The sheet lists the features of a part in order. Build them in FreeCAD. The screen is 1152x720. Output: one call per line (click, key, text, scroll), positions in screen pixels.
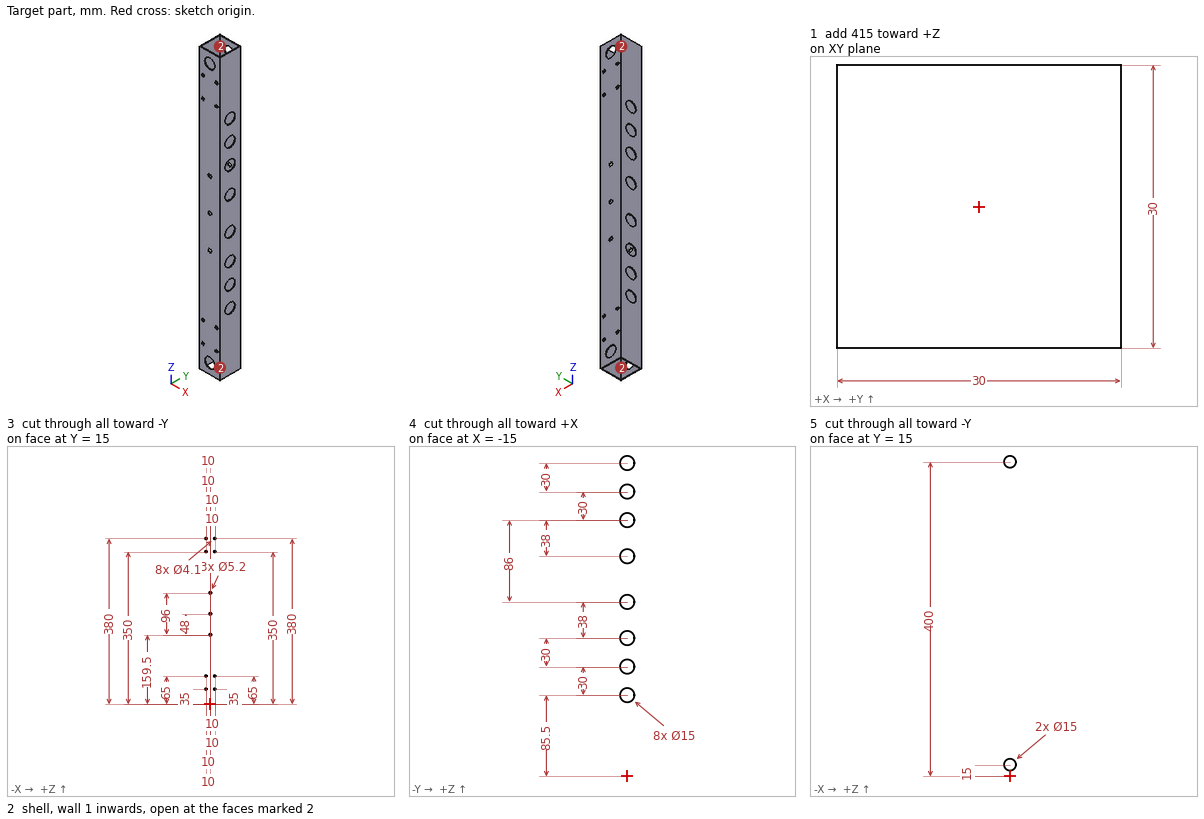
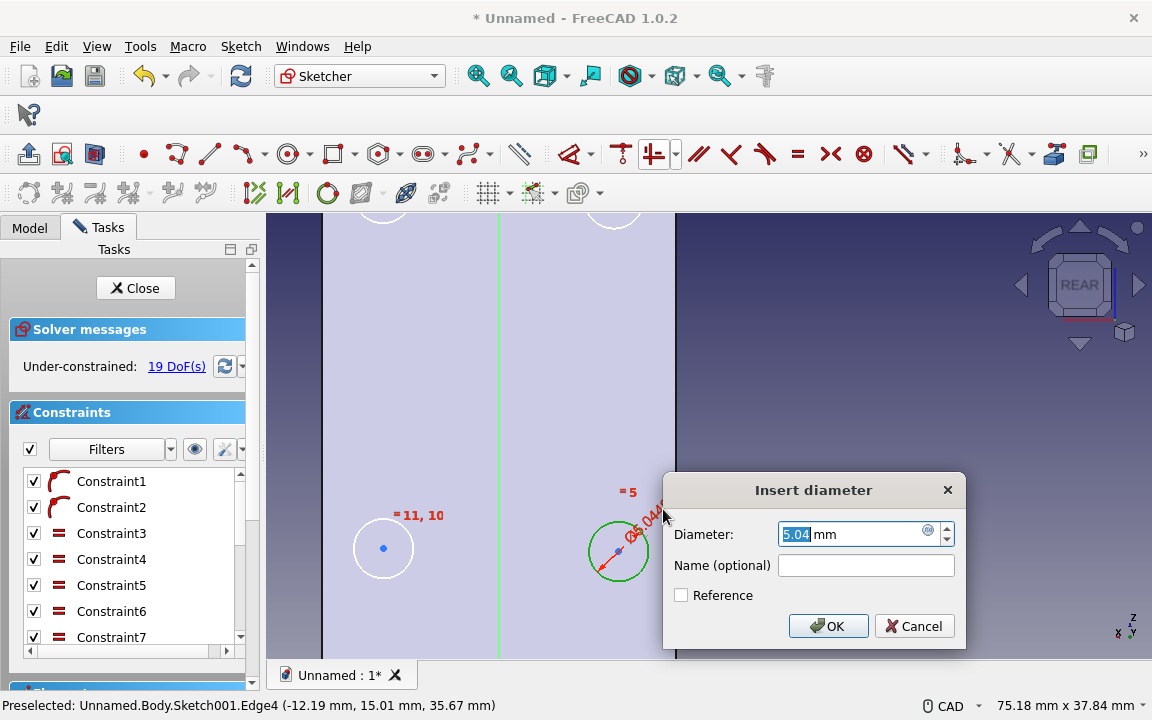
text(4.1)
key(Return)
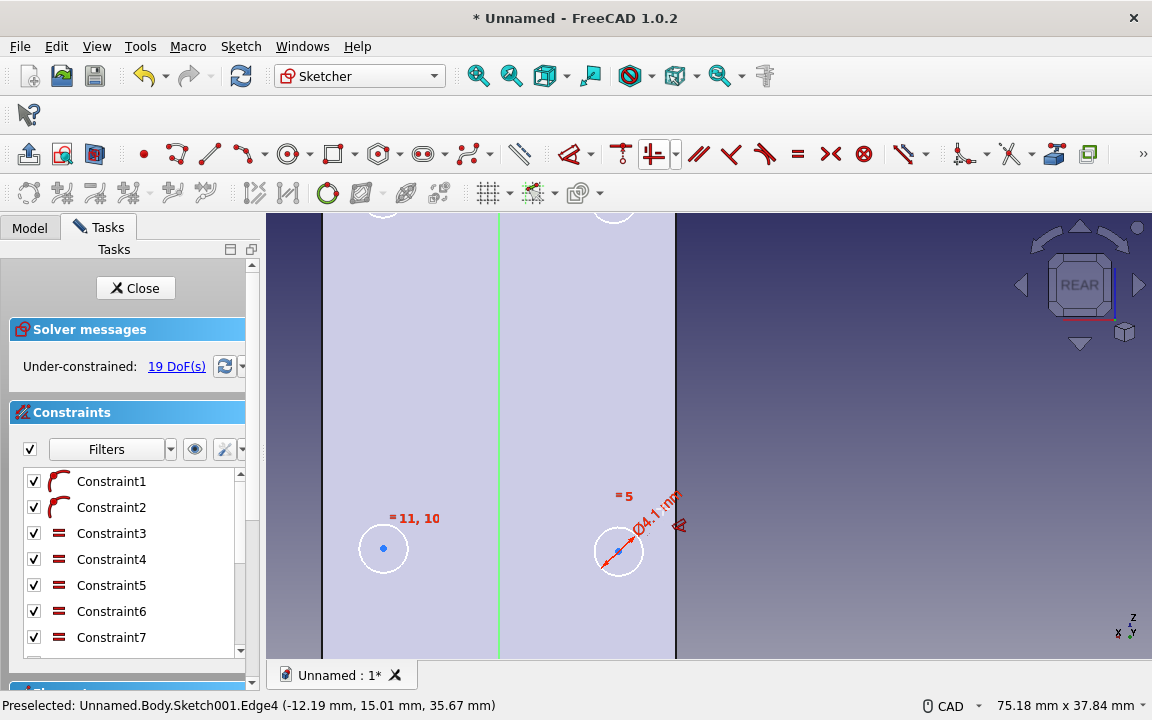
scroll(650, 548, down, 14)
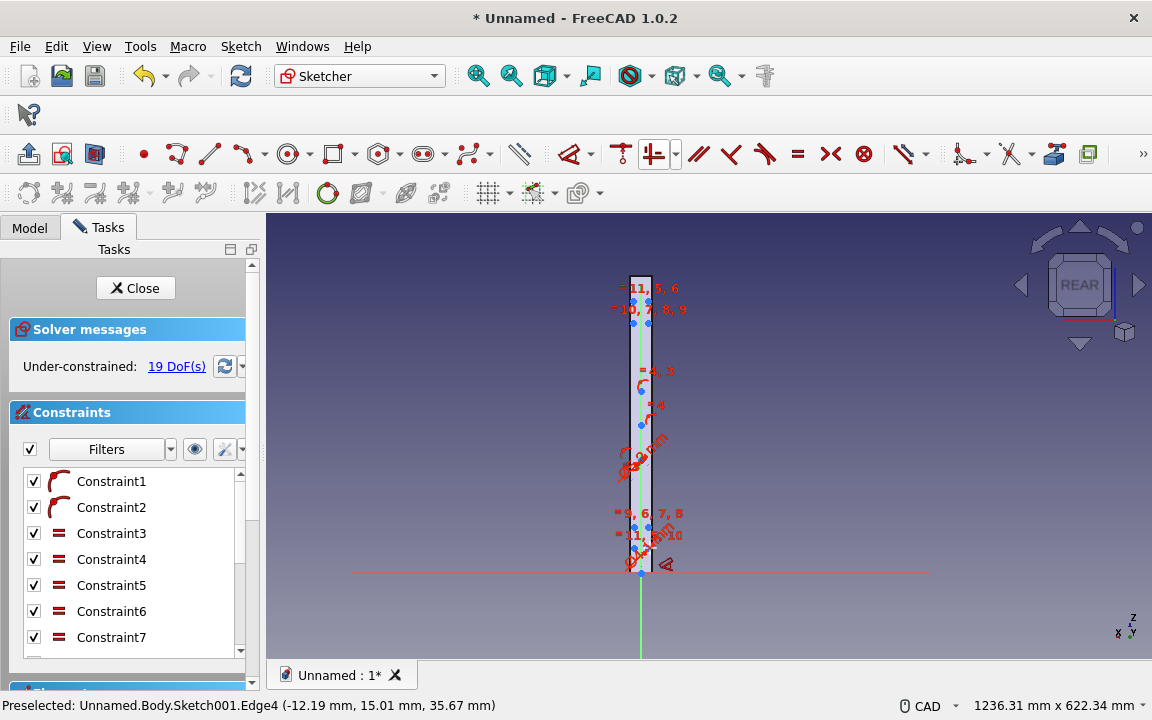
scroll(649, 549, up, 9)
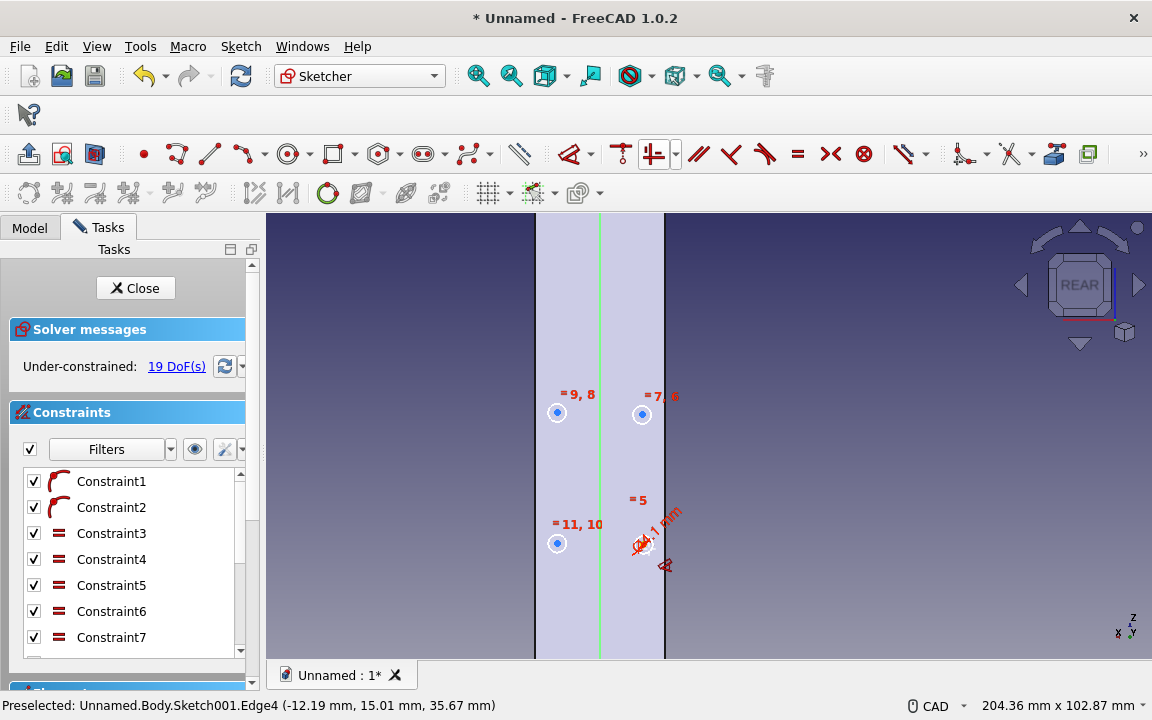
click(644, 545)
click(622, 487)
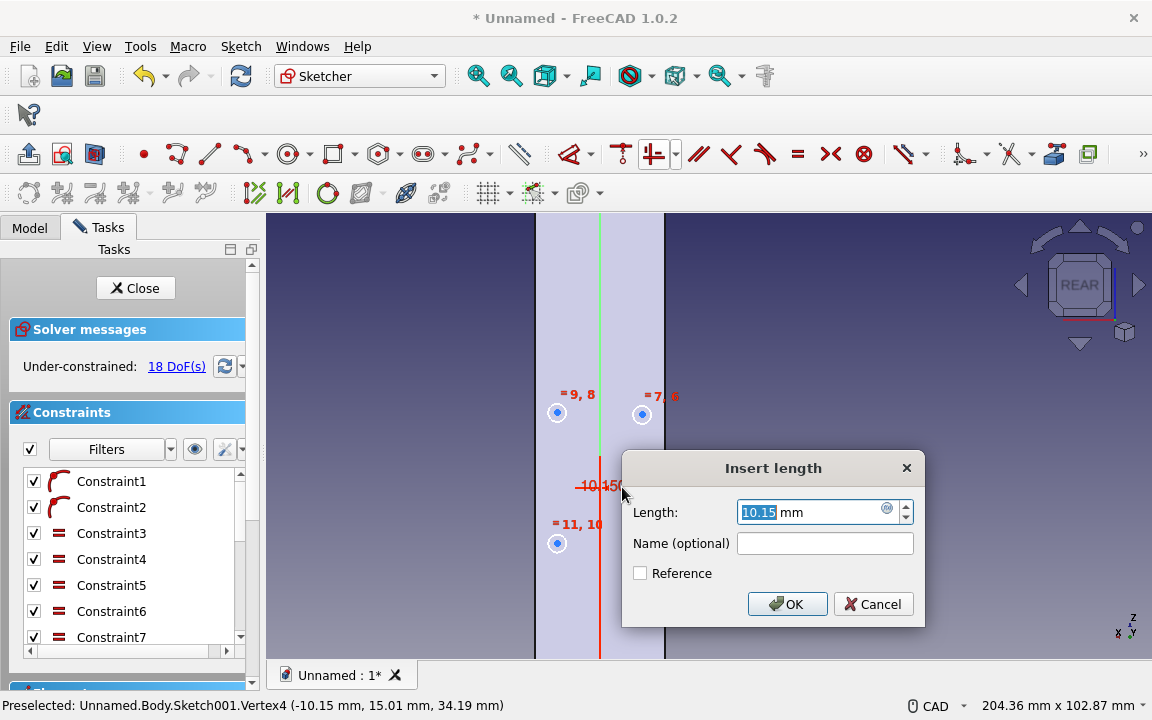
text(10)
key(Return)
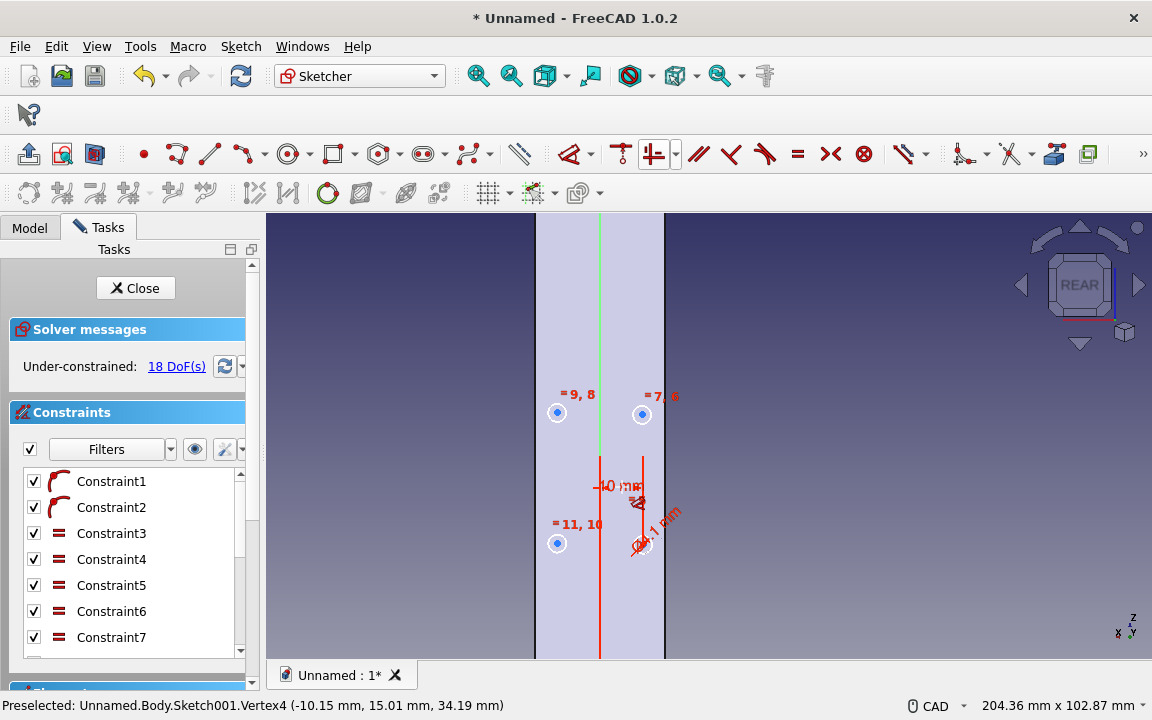
scroll(649, 549, down, 9)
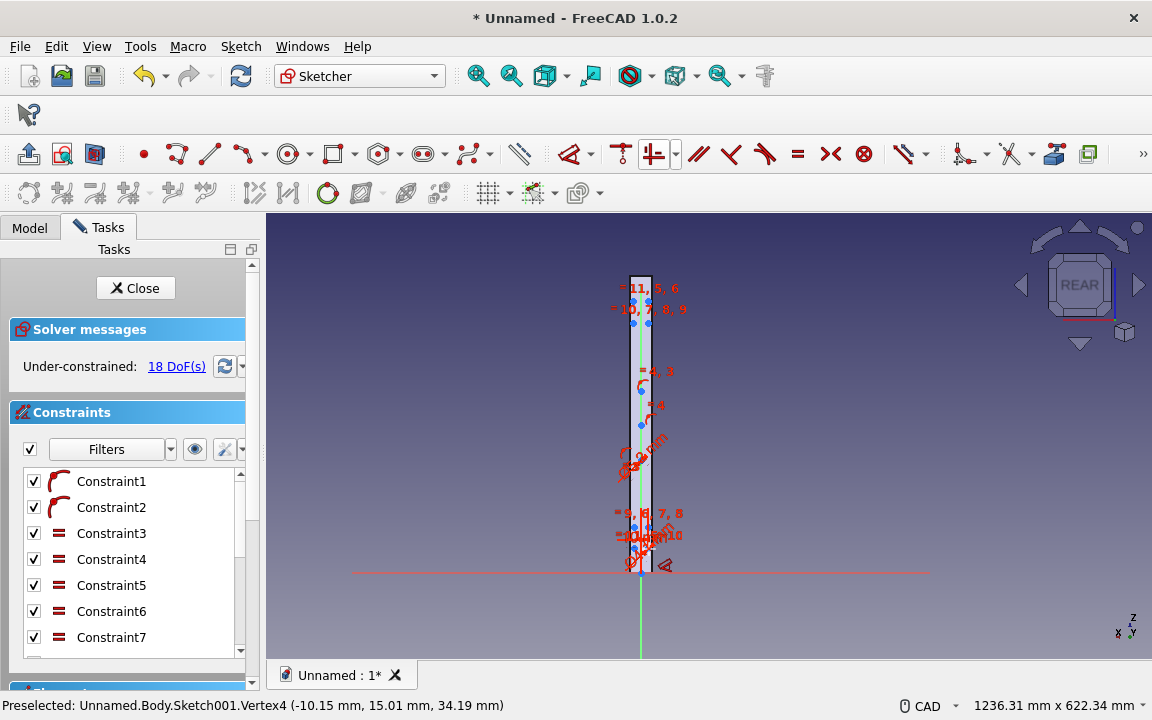
scroll(648, 549, up, 3)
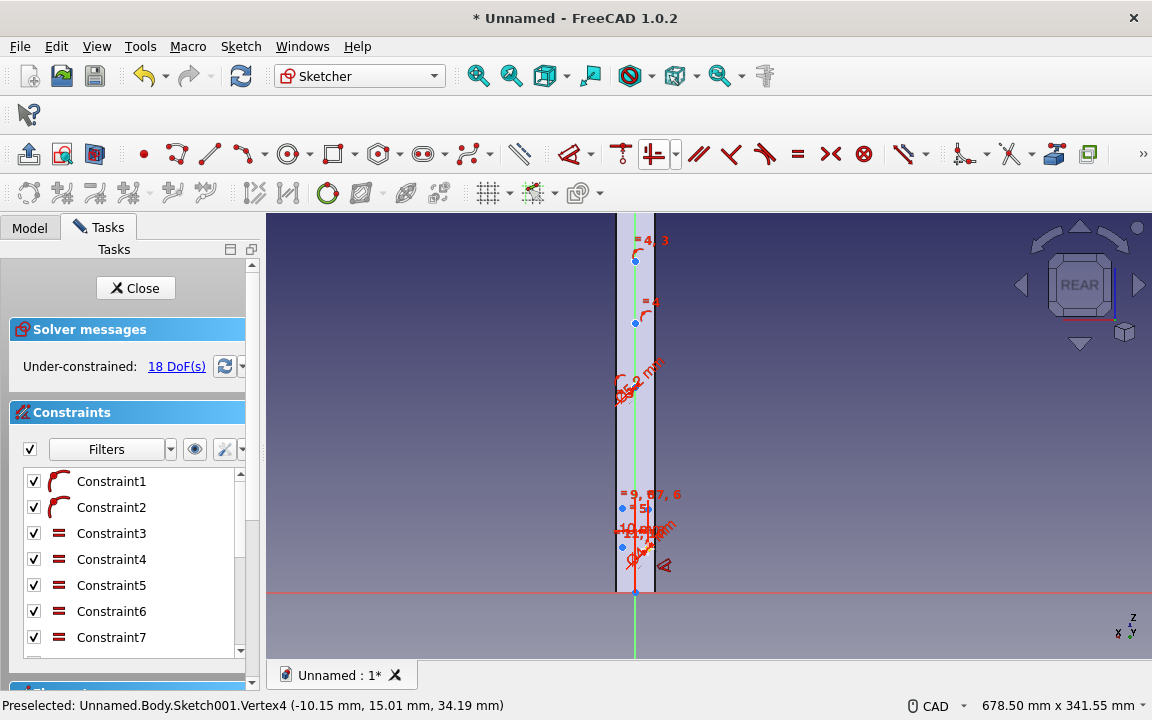
click(648, 548)
click(682, 571)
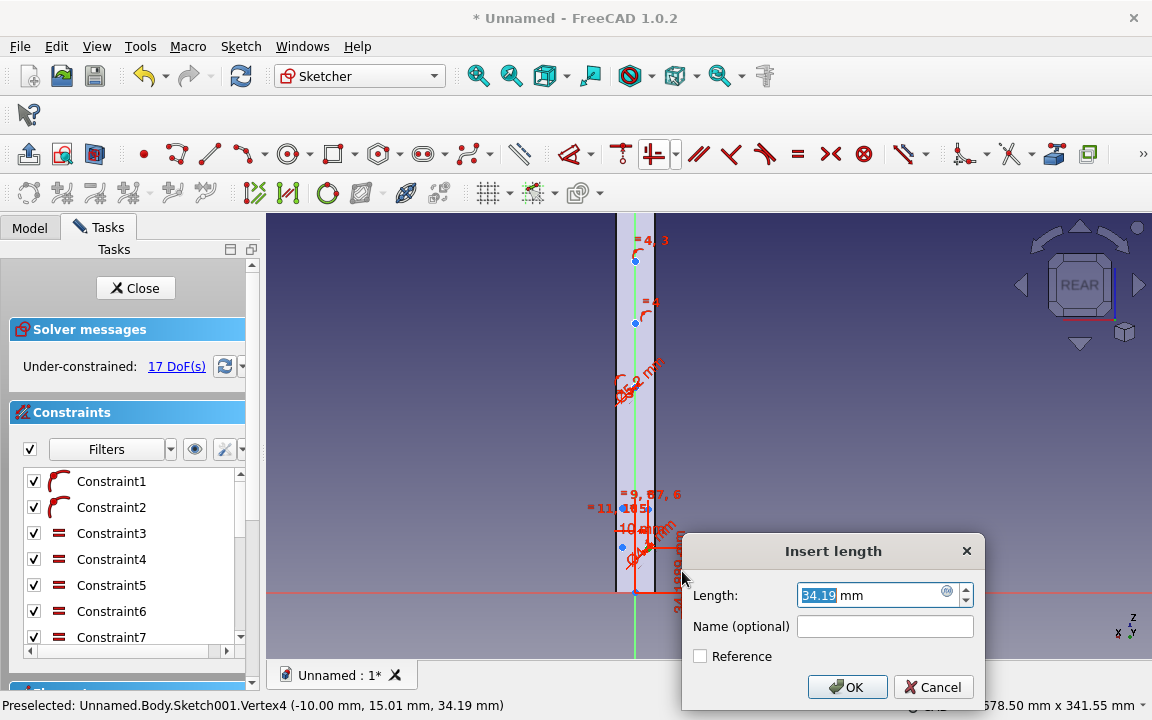
text(35)
key(Return)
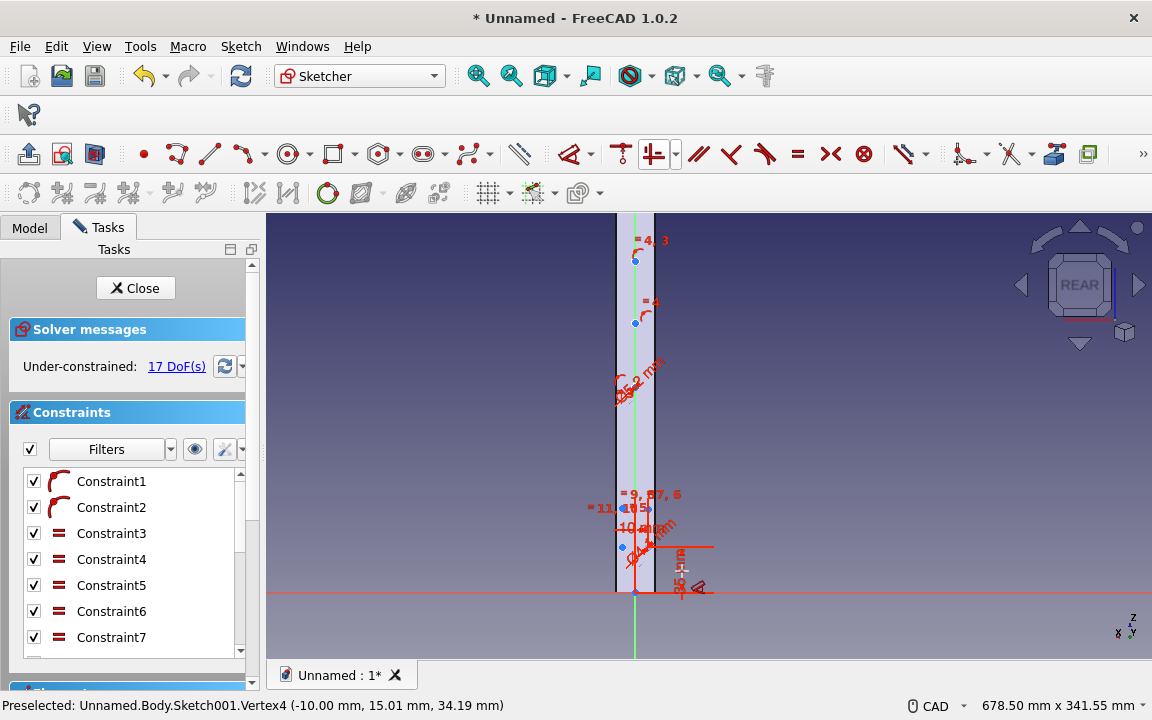
scroll(647, 549, down, 3)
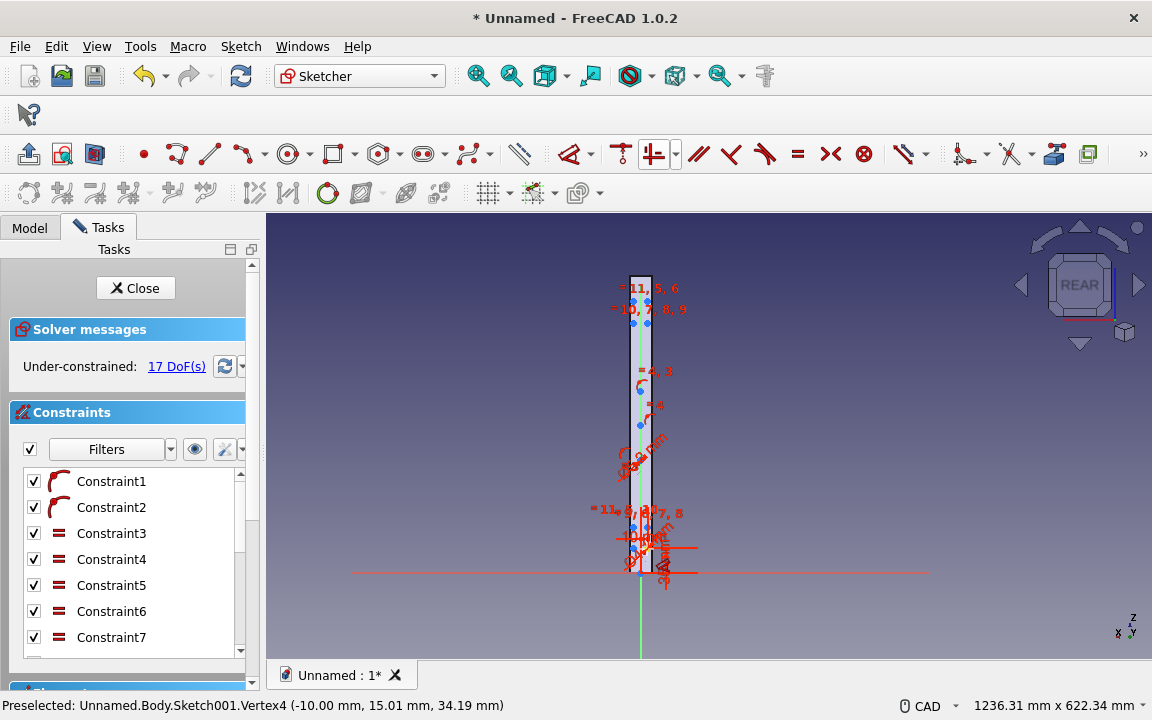
scroll(648, 301, up, 9)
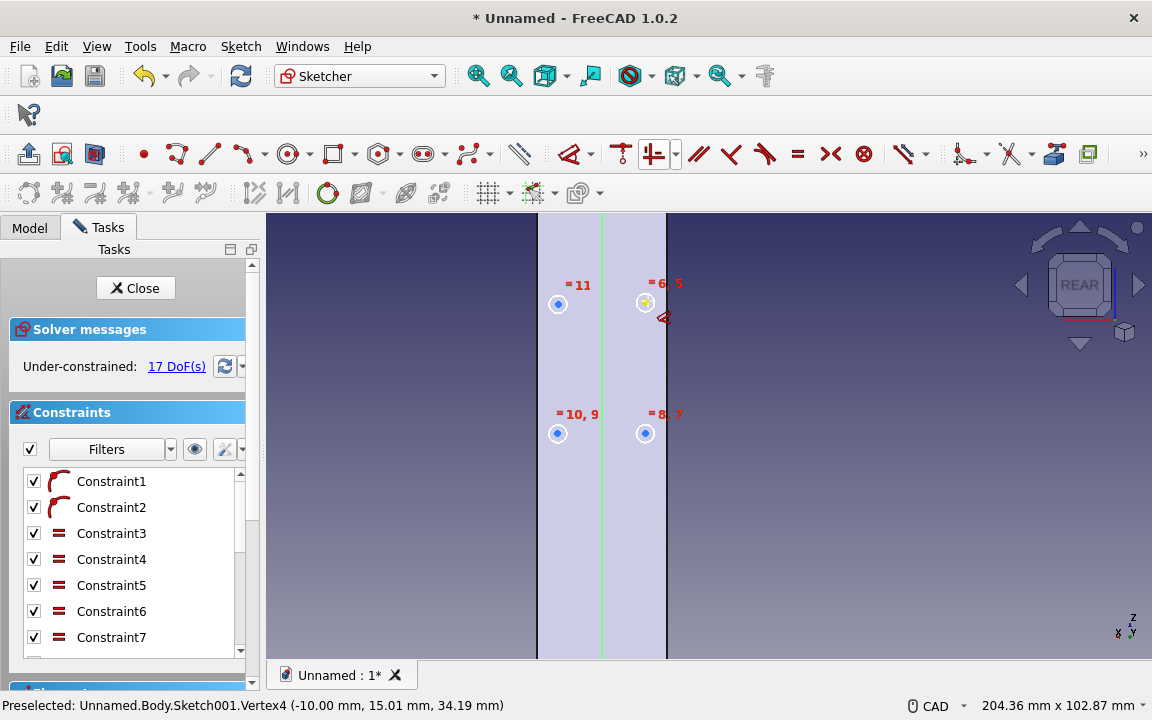
click(646, 303)
click(624, 269)